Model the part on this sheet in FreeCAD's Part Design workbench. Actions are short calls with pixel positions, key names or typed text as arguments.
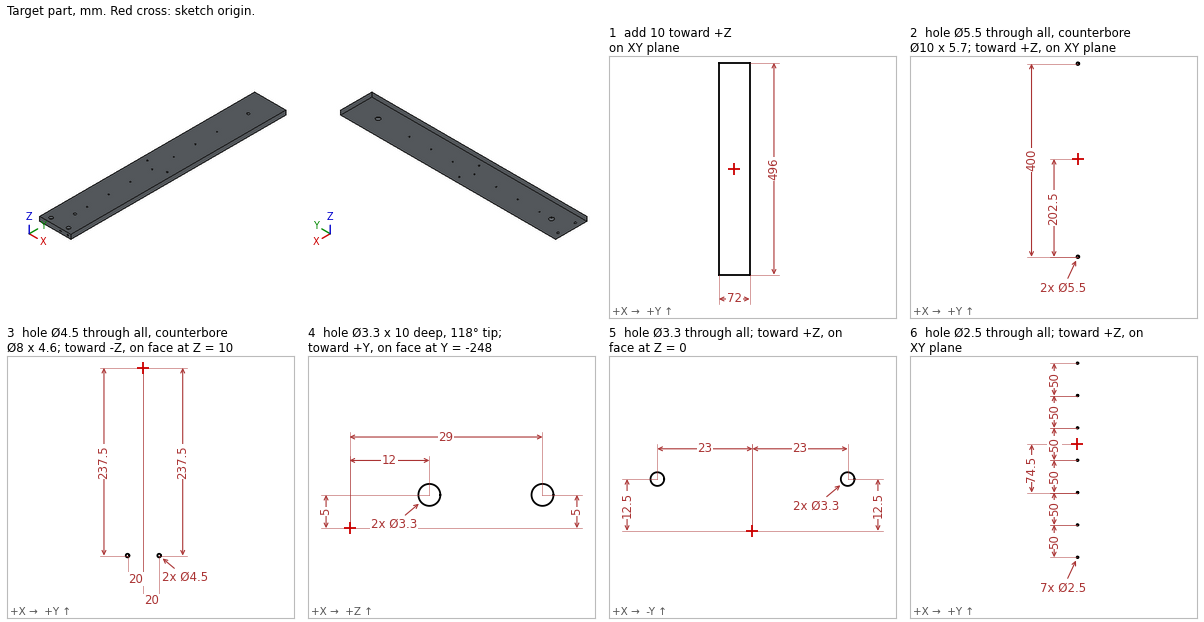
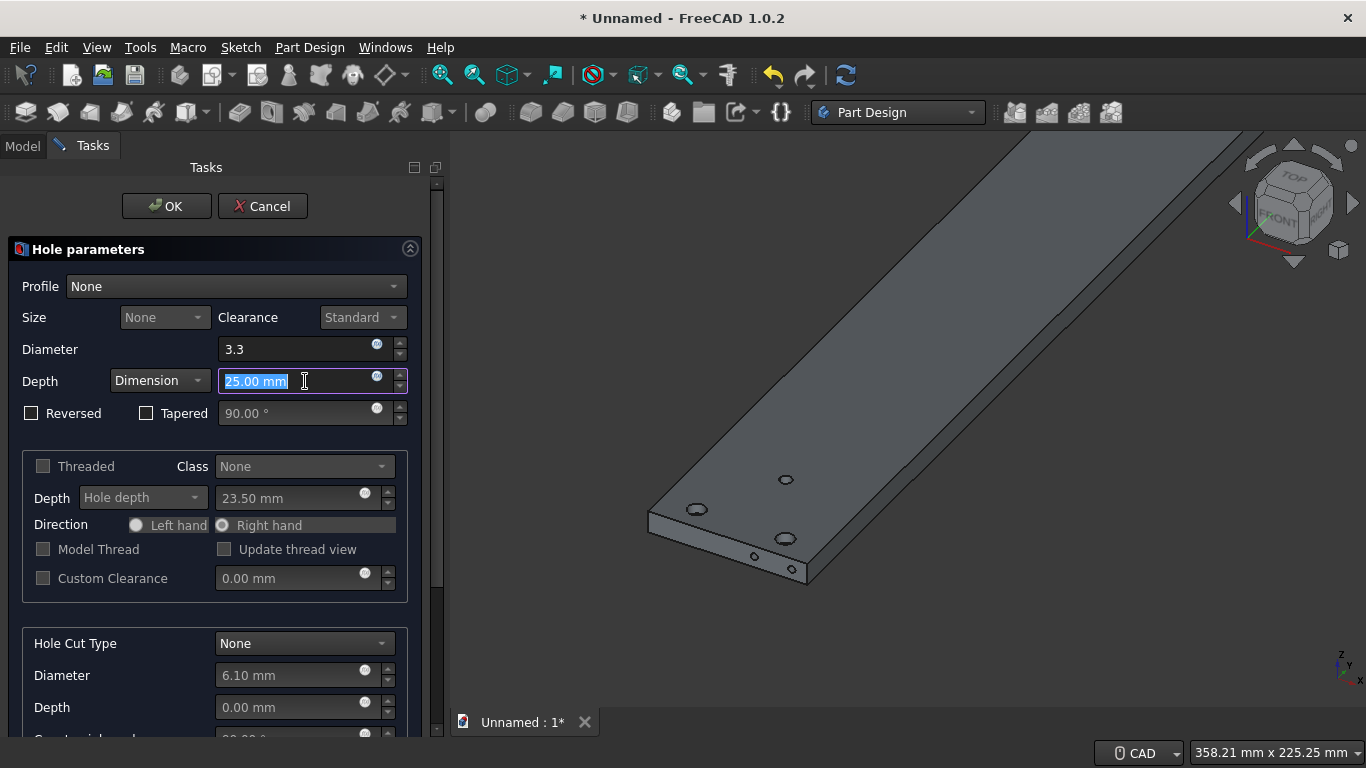
text(10)
key(Tab)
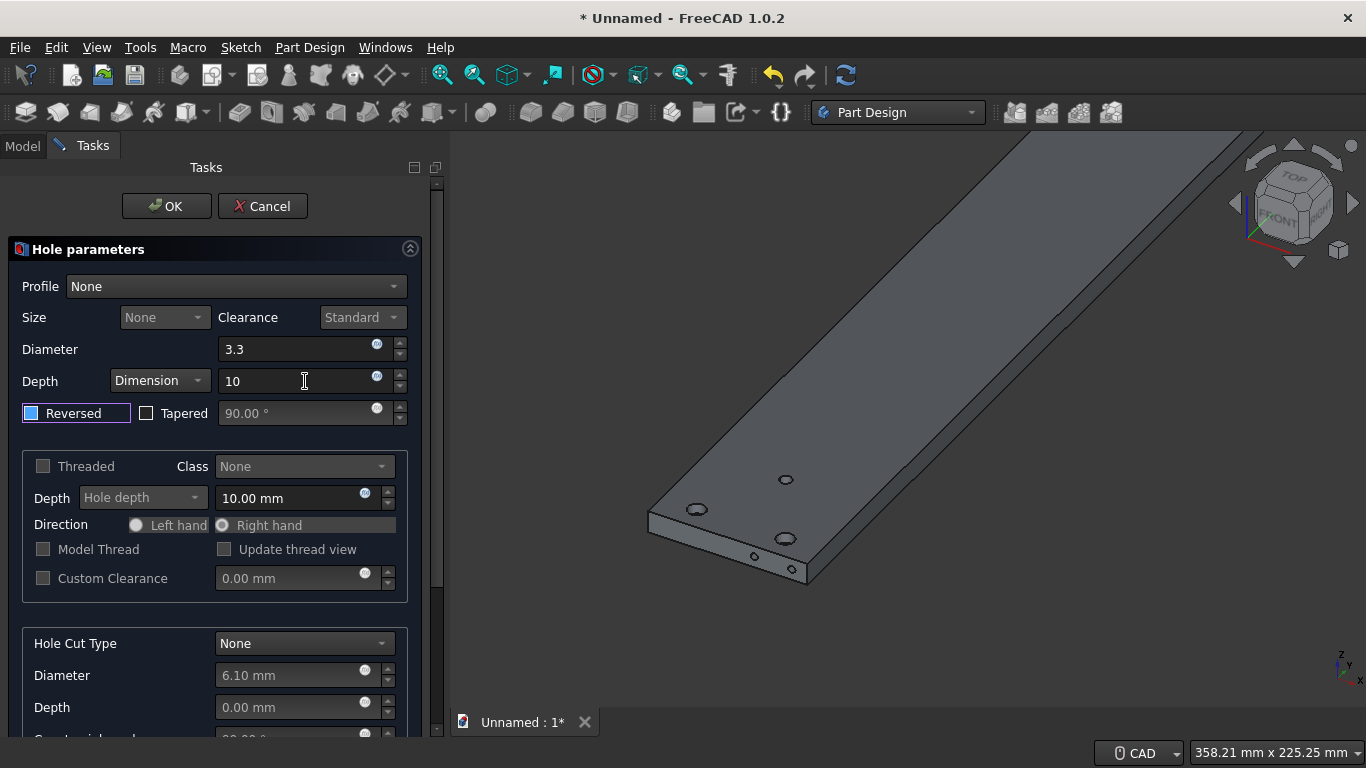
click(167, 206)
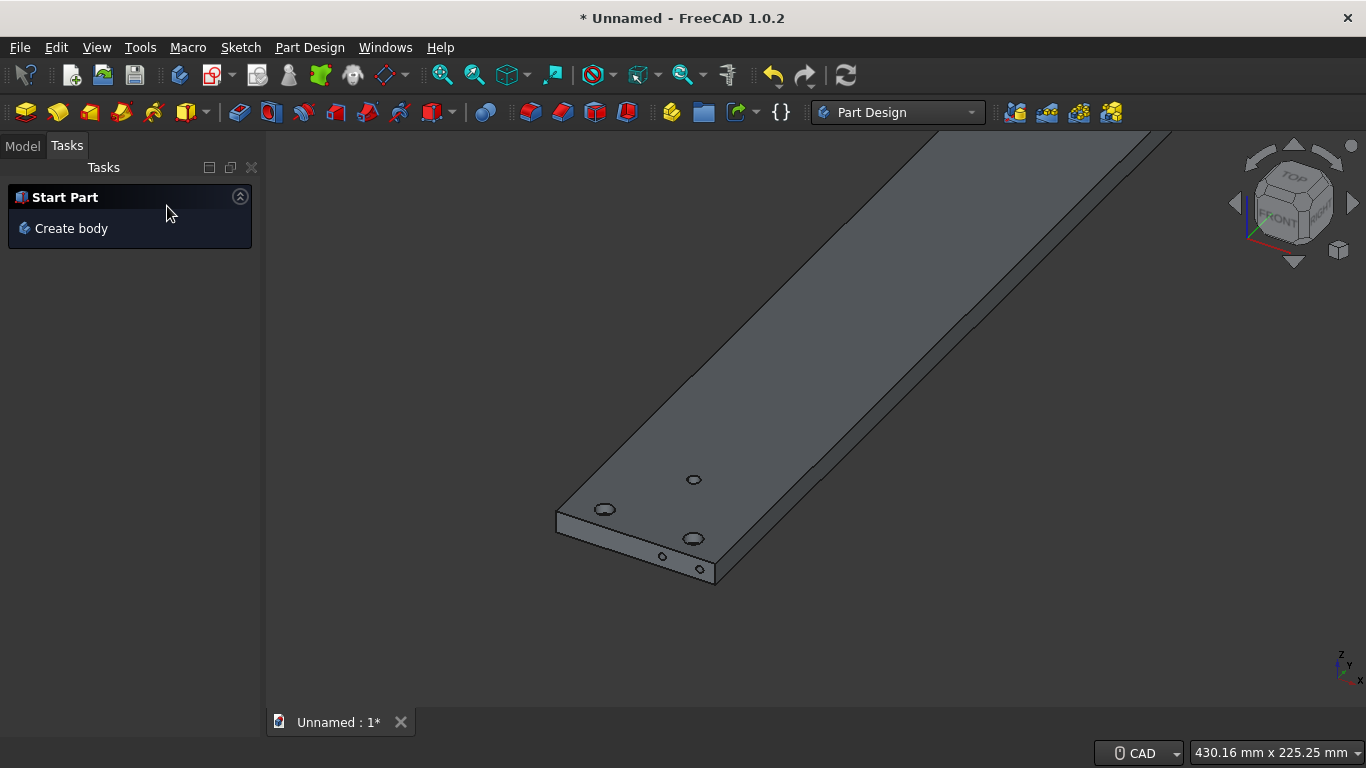
key(v)
key(f)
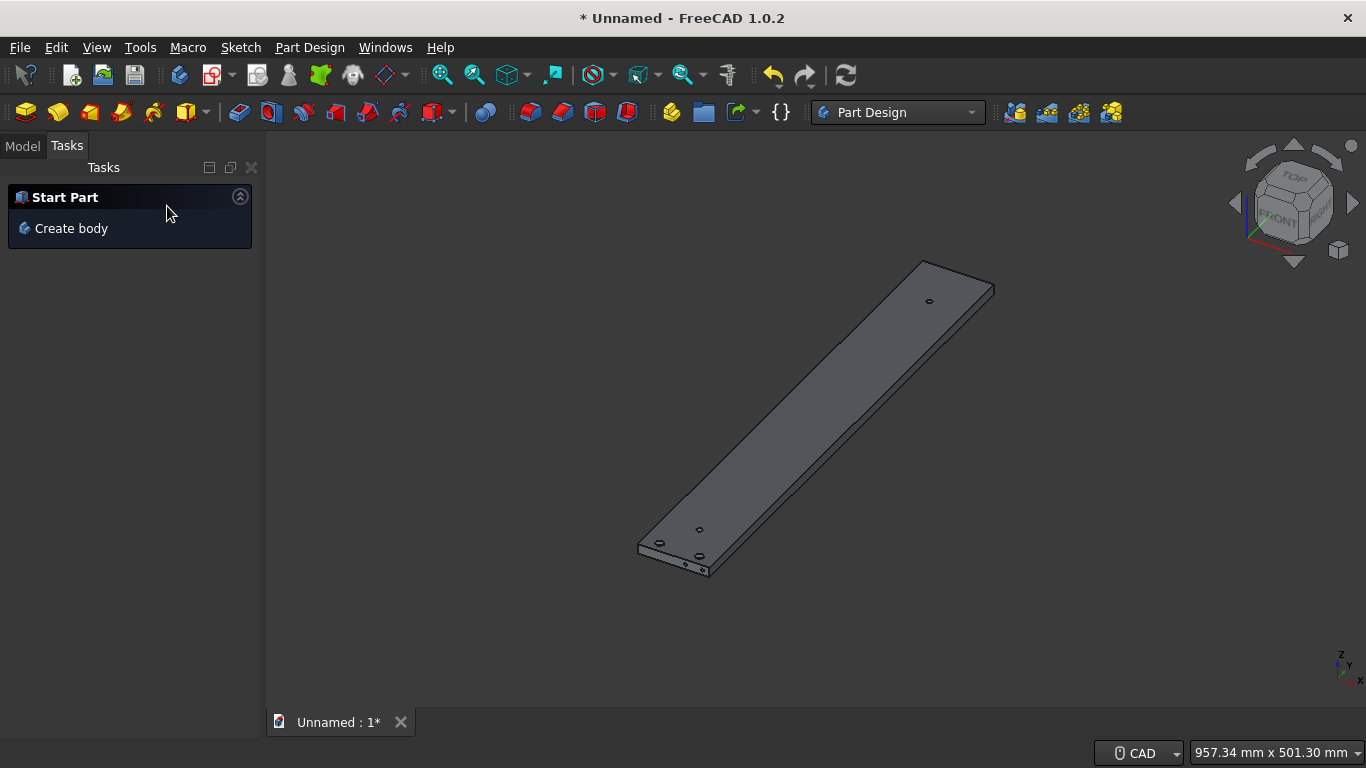
key(5)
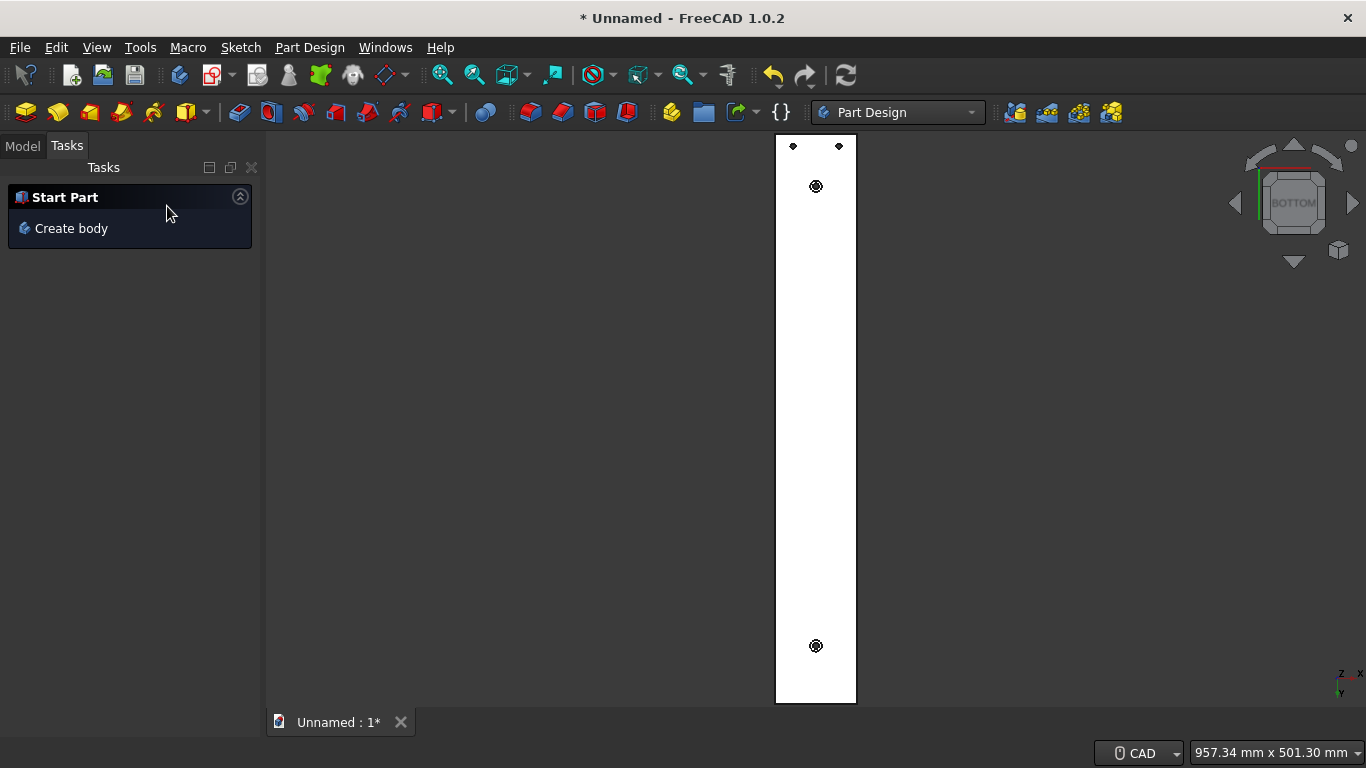
click(816, 581)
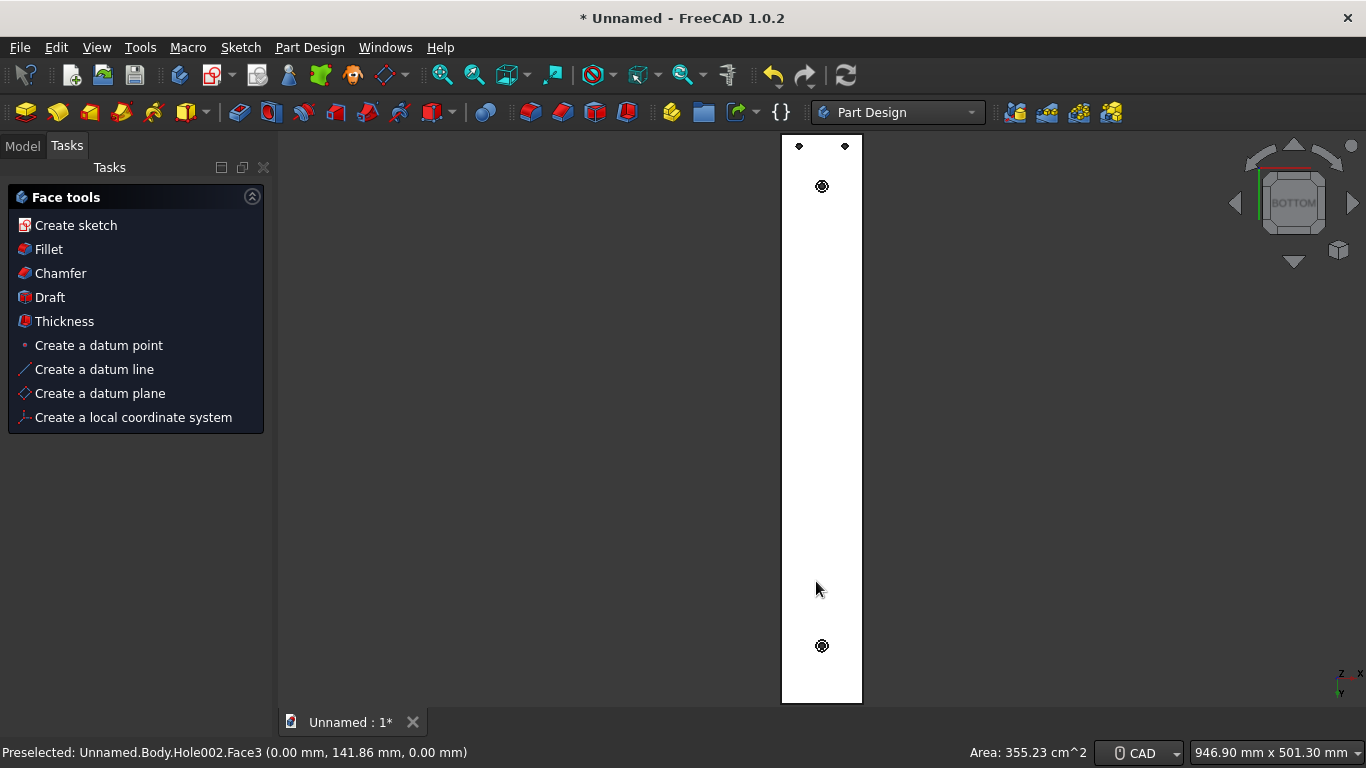
click(212, 76)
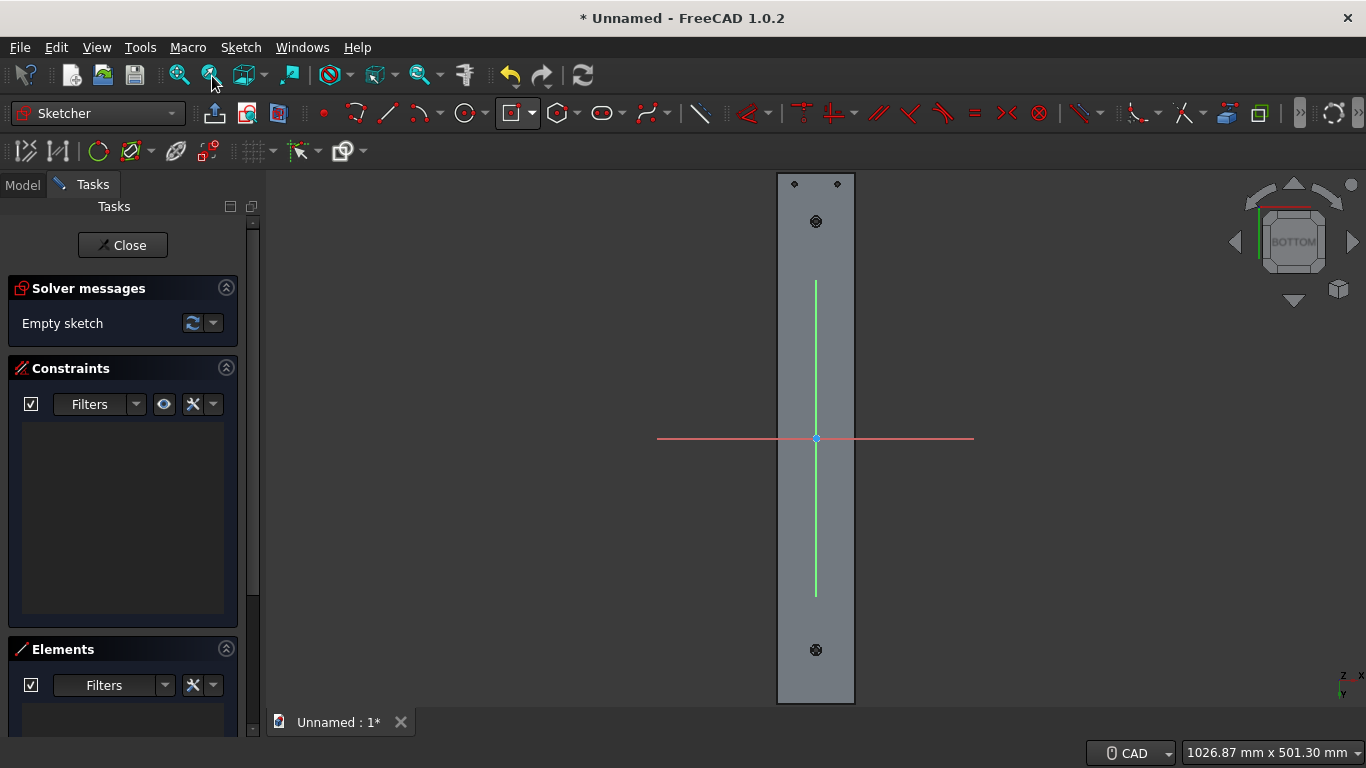
scroll(823, 430, up, 12)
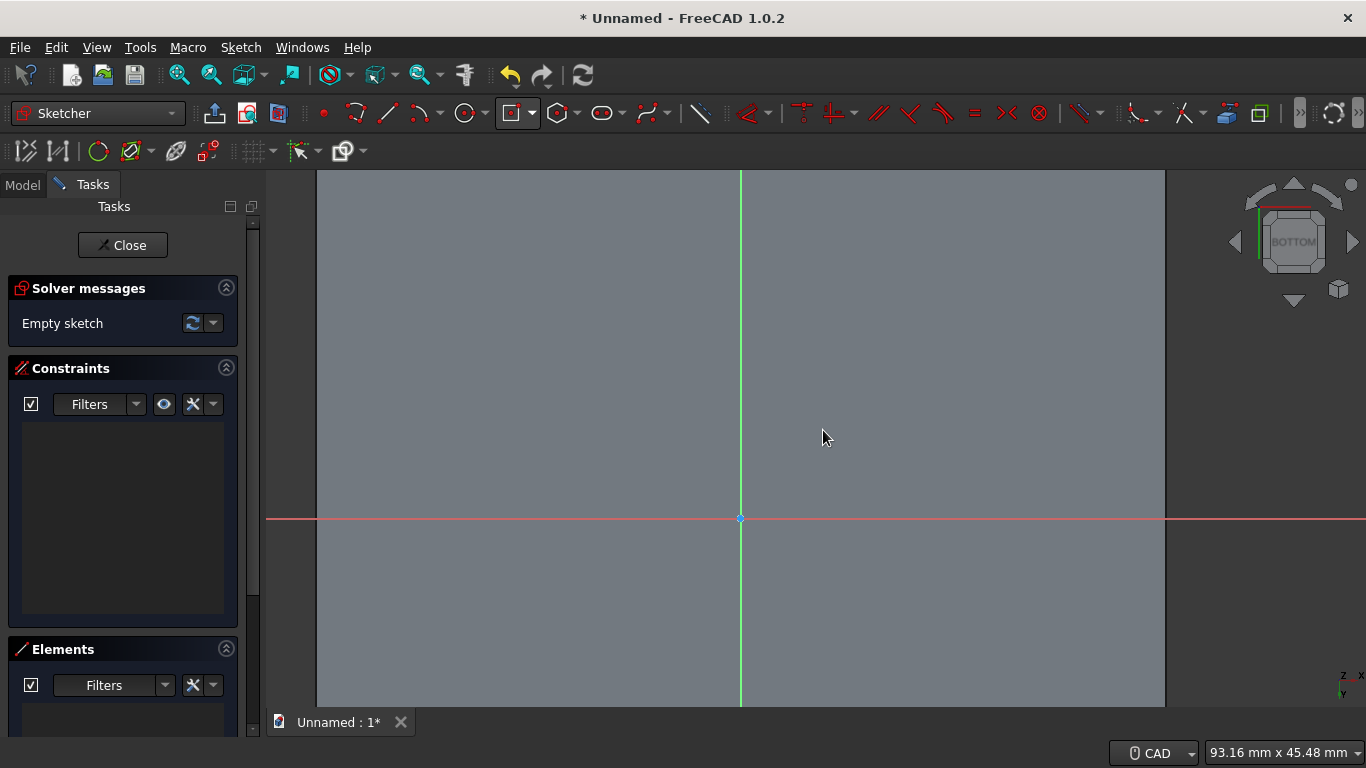
click(466, 114)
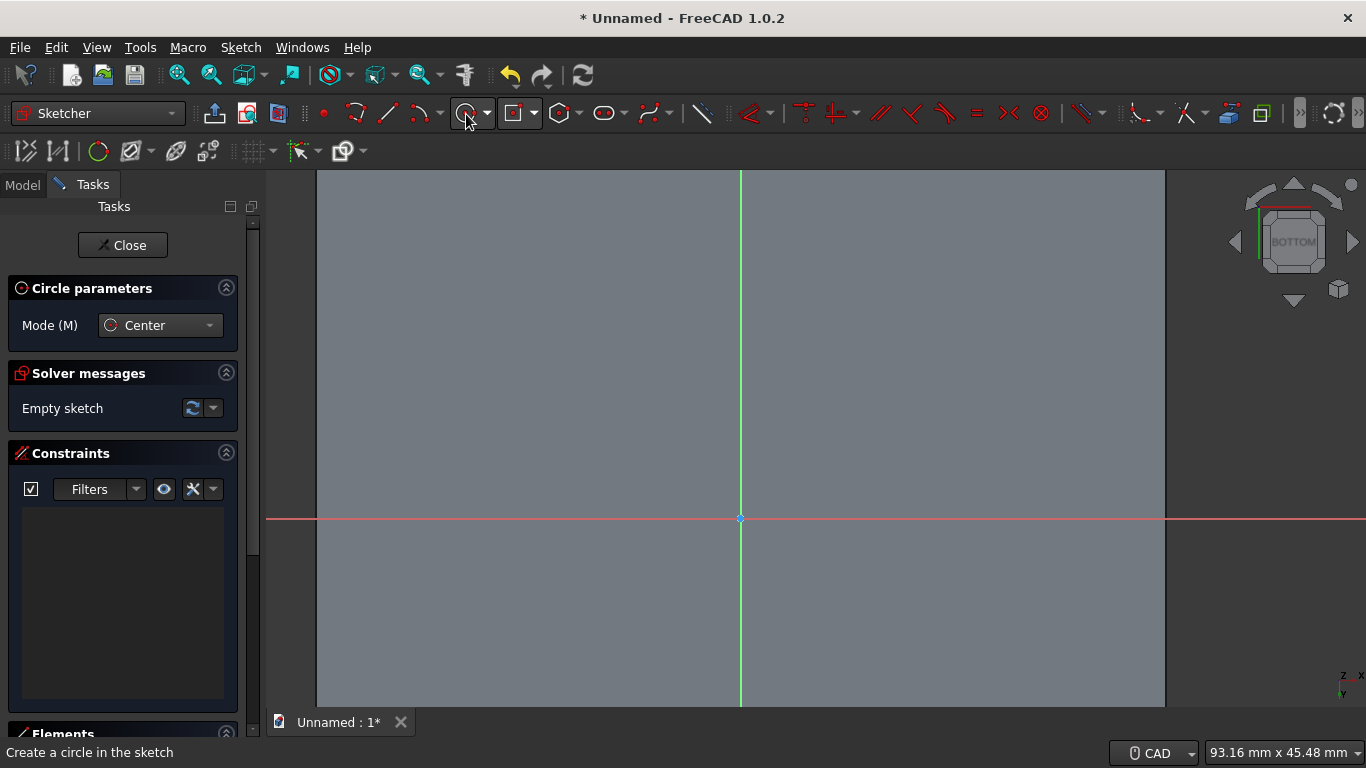
click(1012, 371)
click(1026, 357)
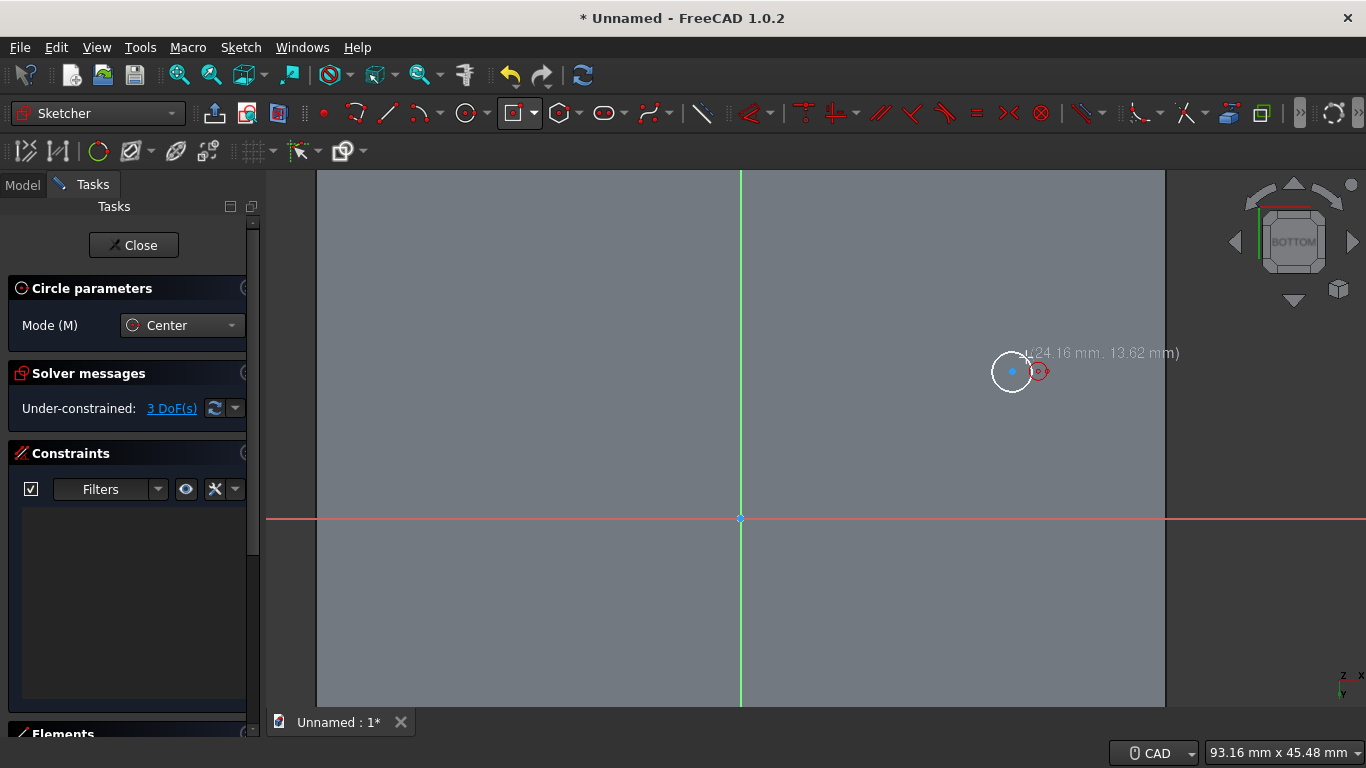
click(469, 371)
click(483, 357)
key(Escape)